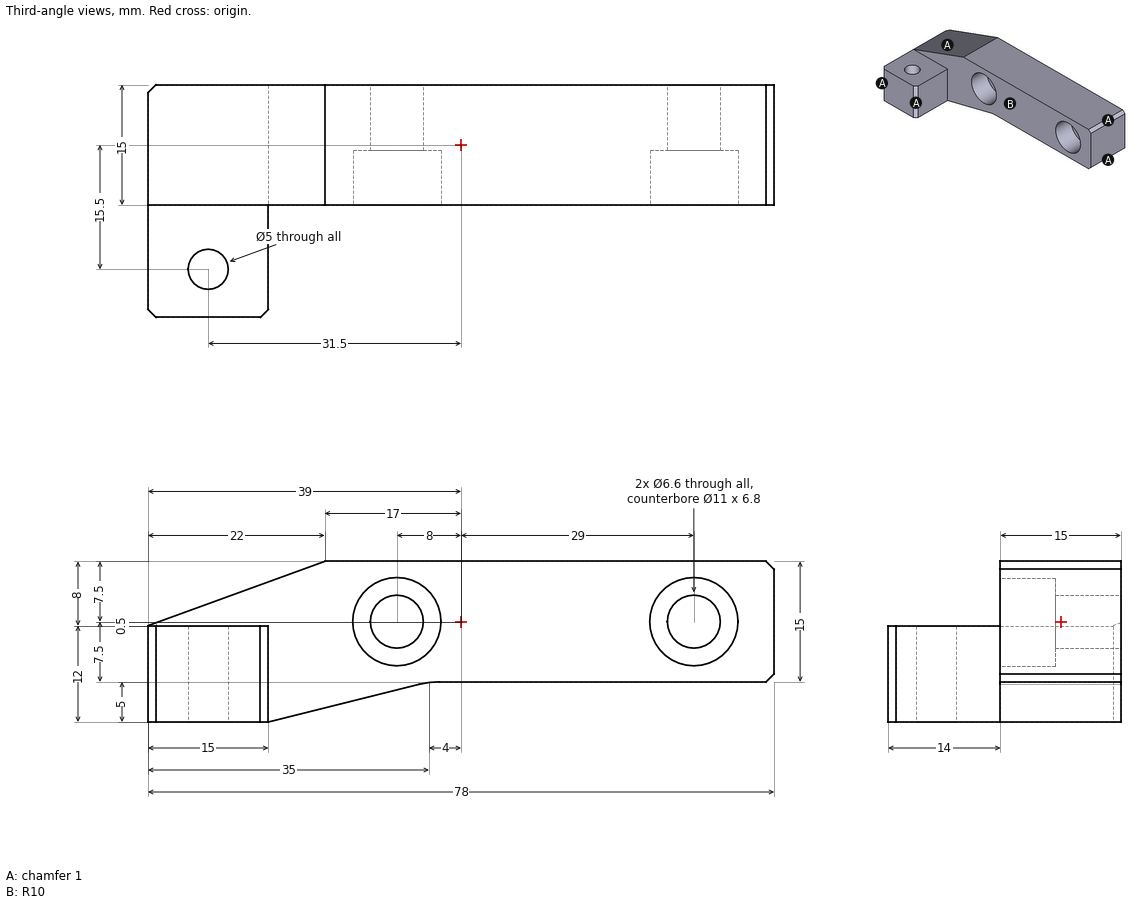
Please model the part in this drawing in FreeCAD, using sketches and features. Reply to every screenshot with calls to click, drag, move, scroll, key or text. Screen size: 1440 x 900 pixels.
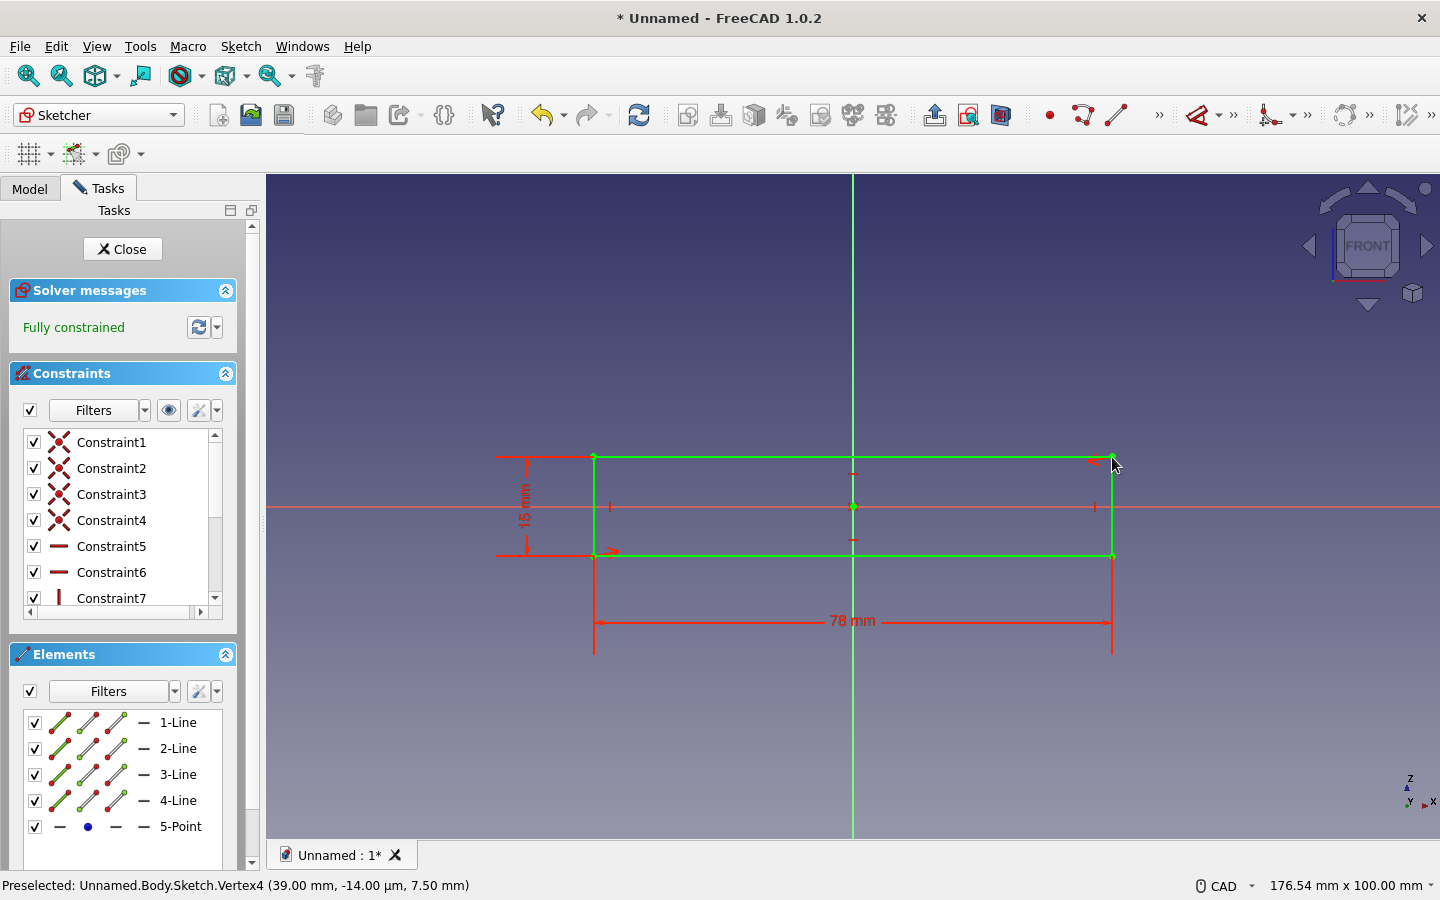
click(123, 249)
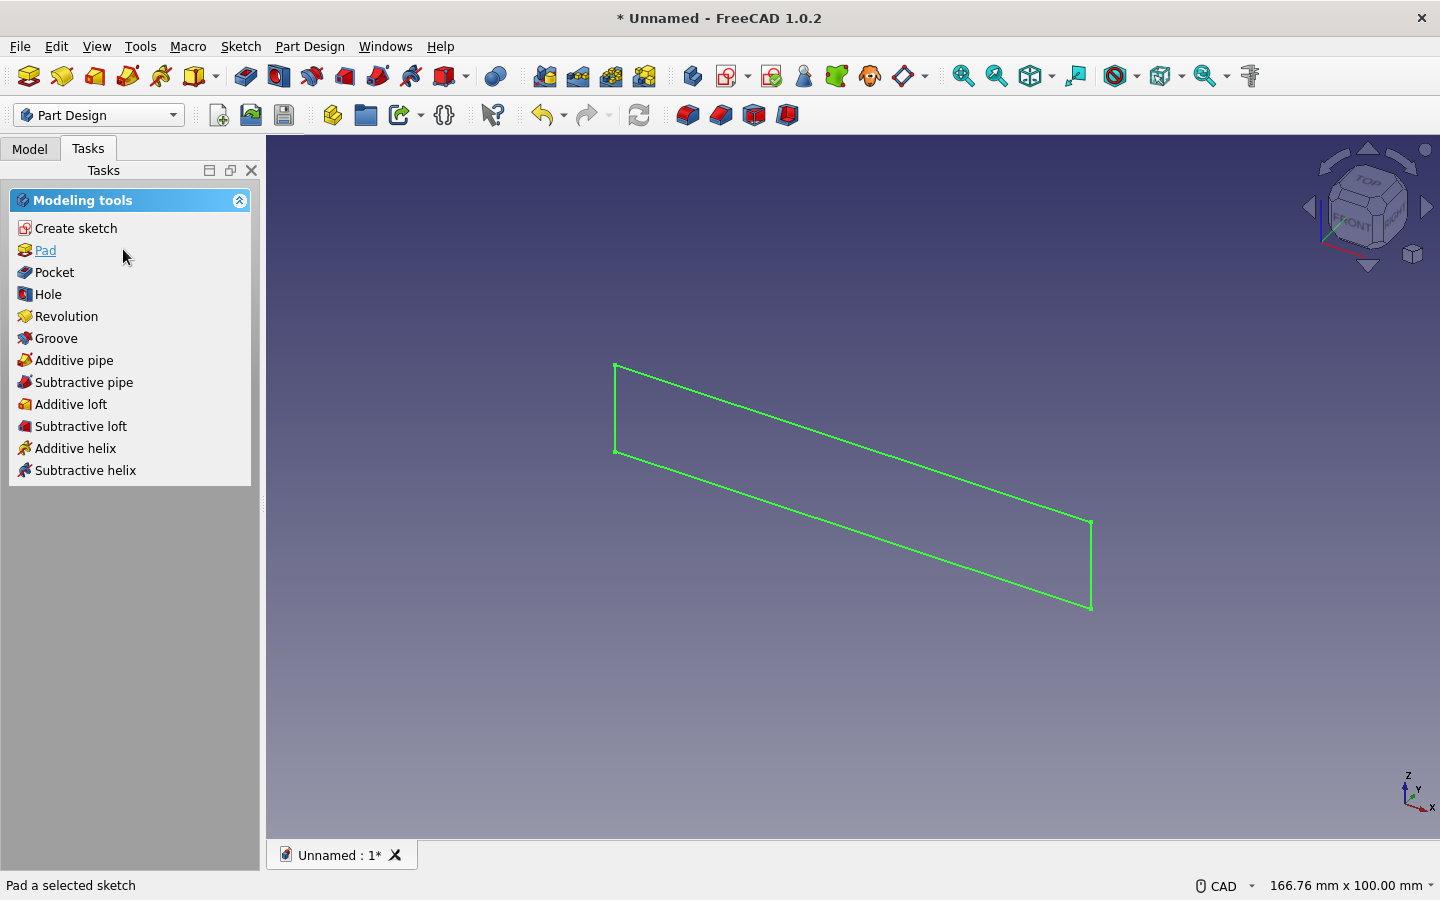
click(29, 76)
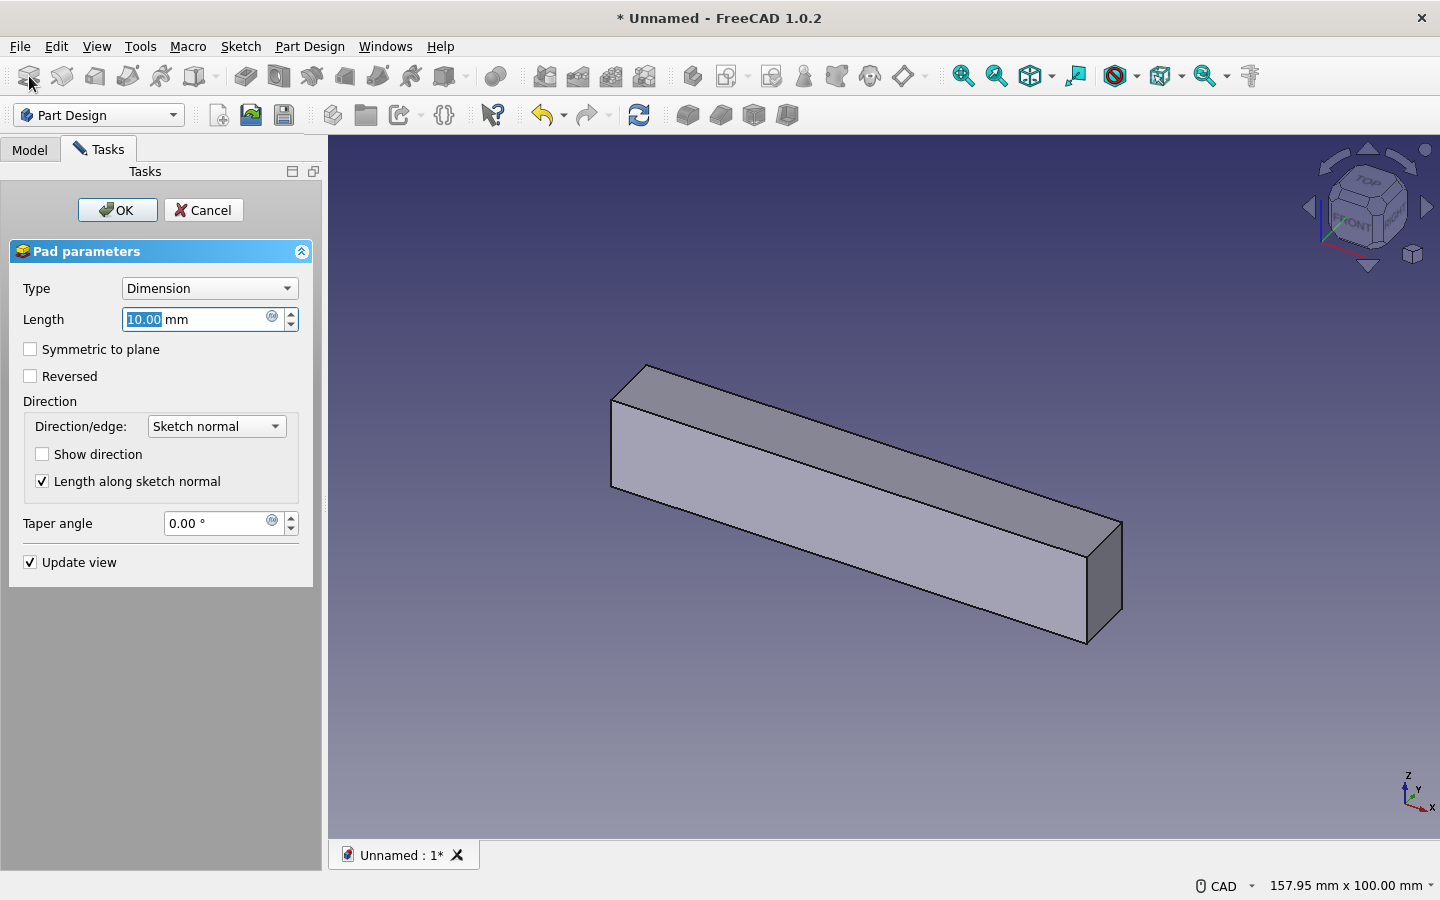
text(15)
key(Tab)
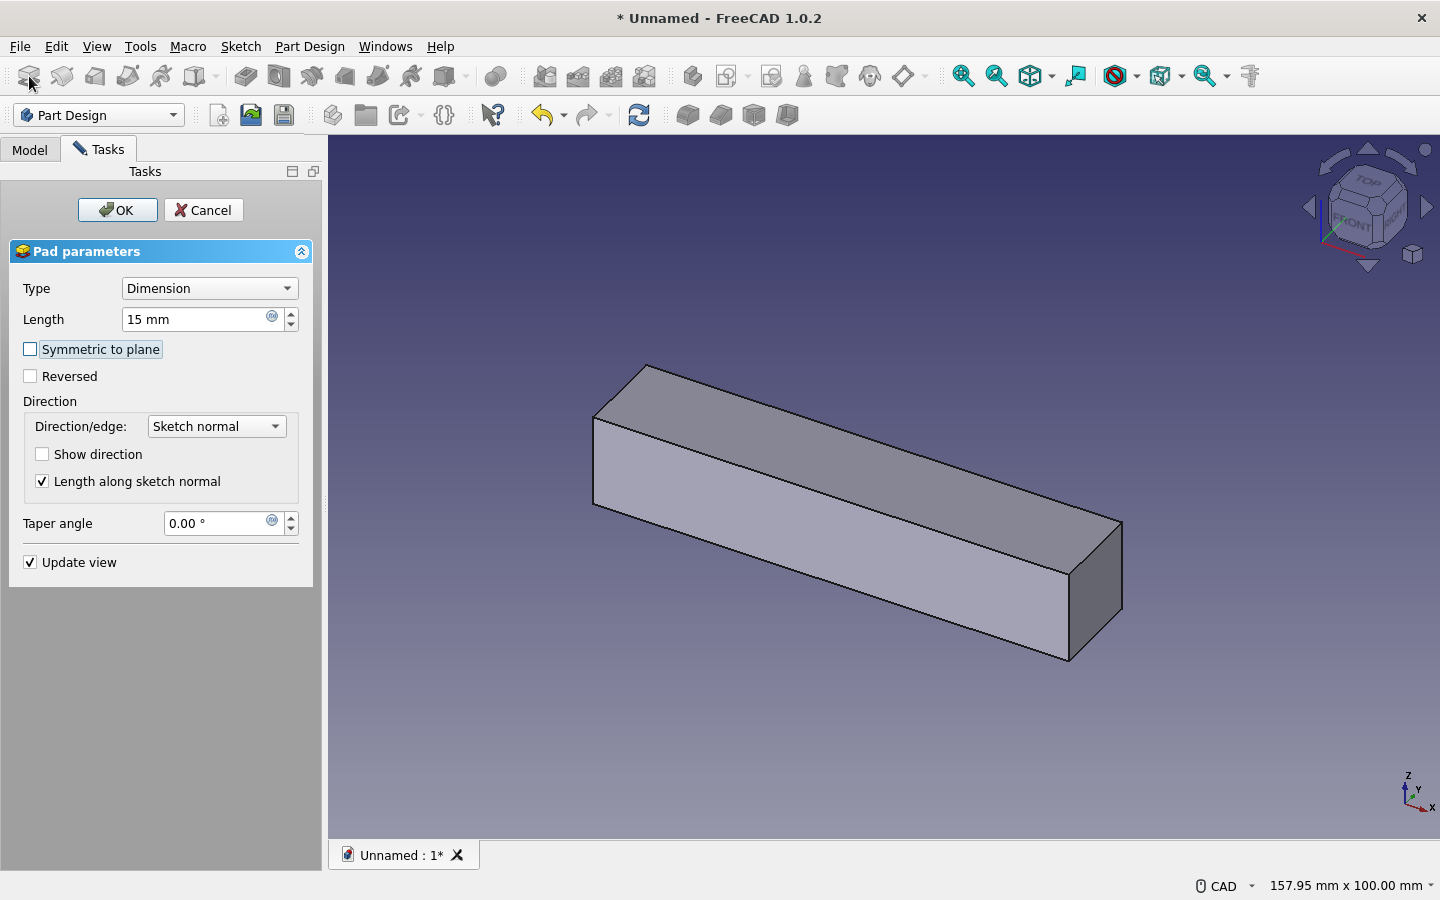
click(31, 349)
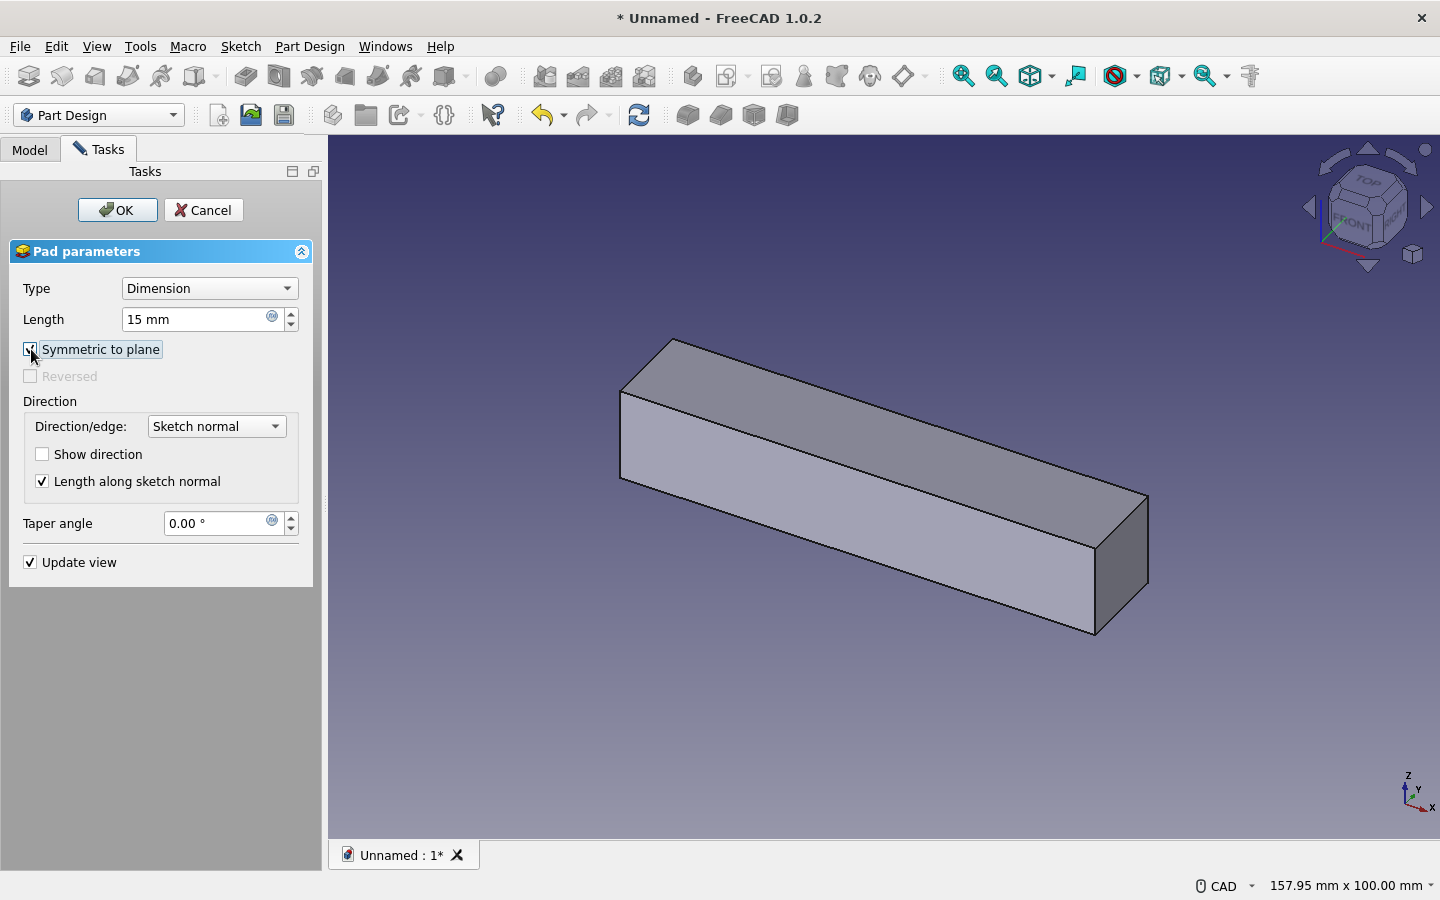
click(118, 210)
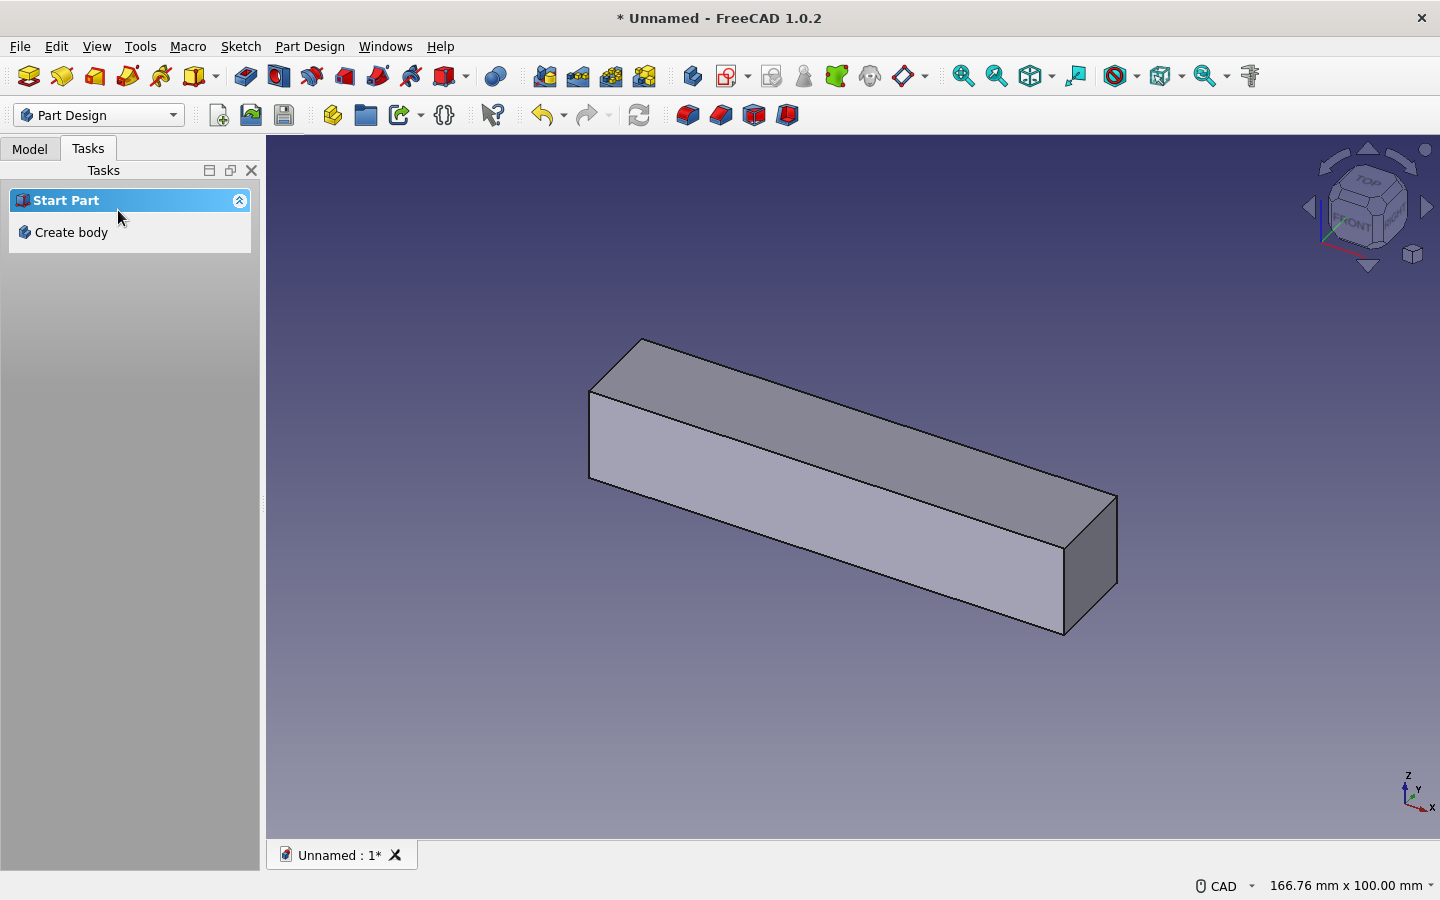
key(v)
key(f)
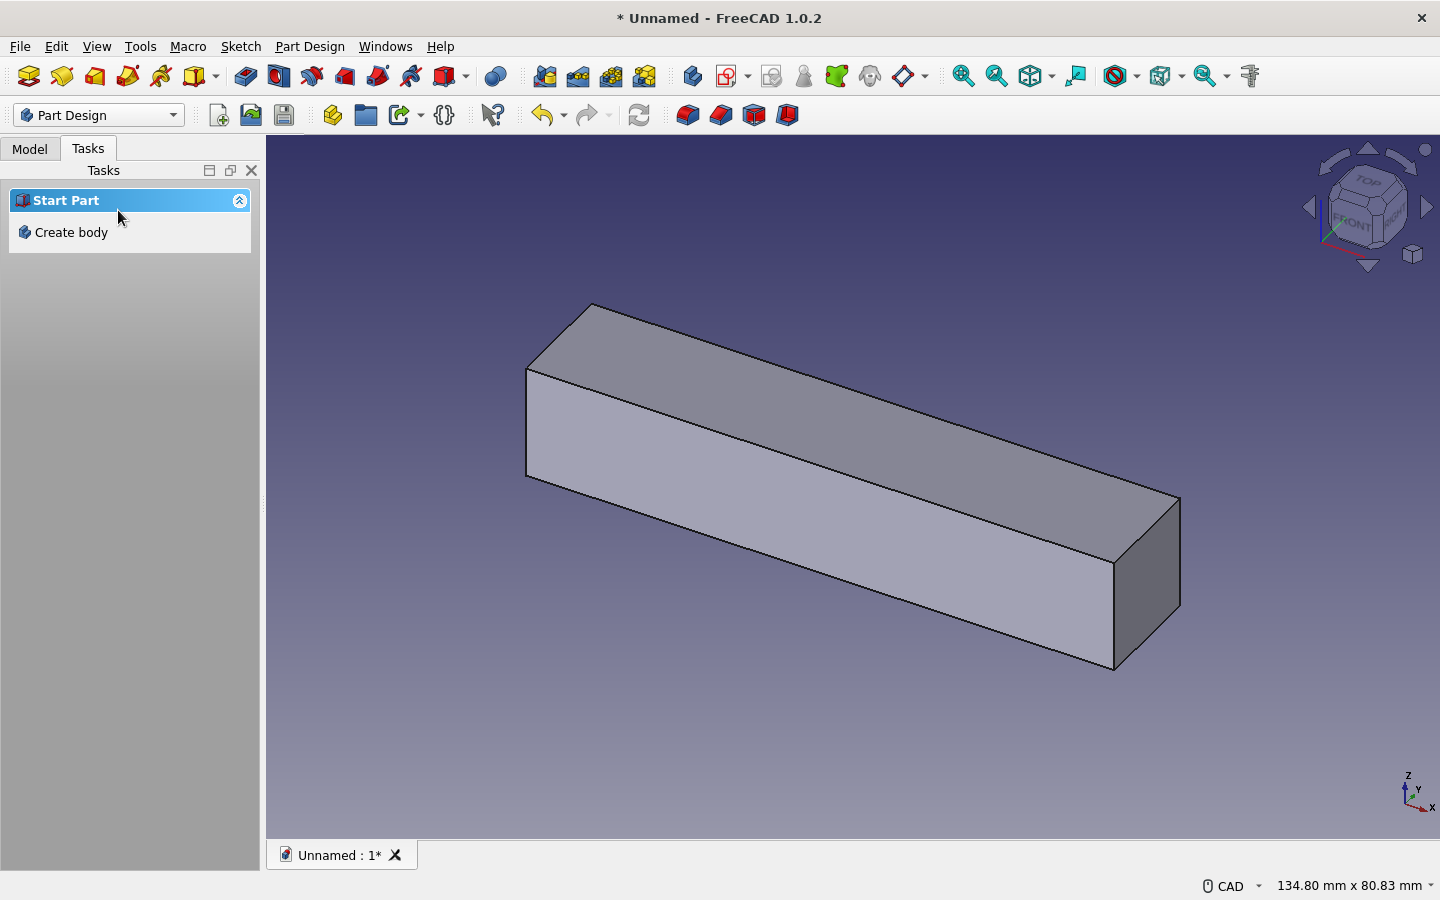
click(988, 574)